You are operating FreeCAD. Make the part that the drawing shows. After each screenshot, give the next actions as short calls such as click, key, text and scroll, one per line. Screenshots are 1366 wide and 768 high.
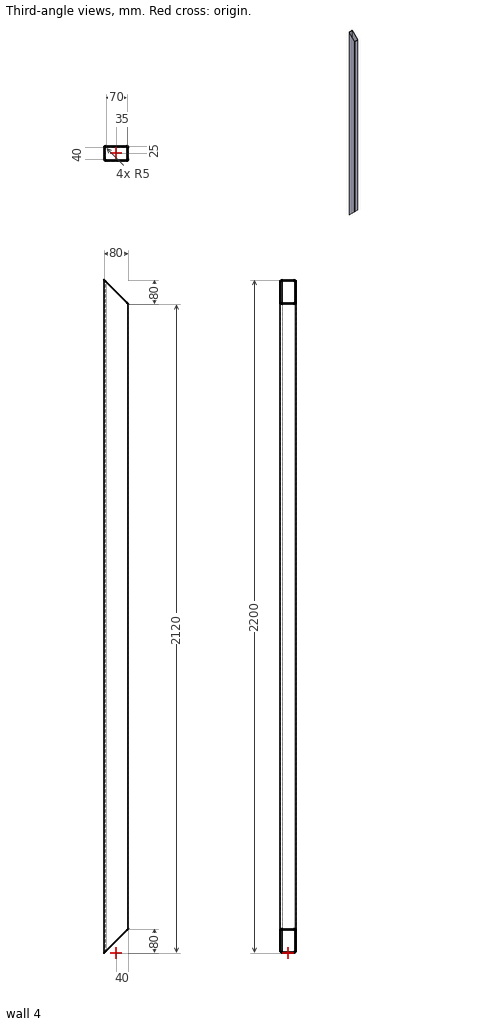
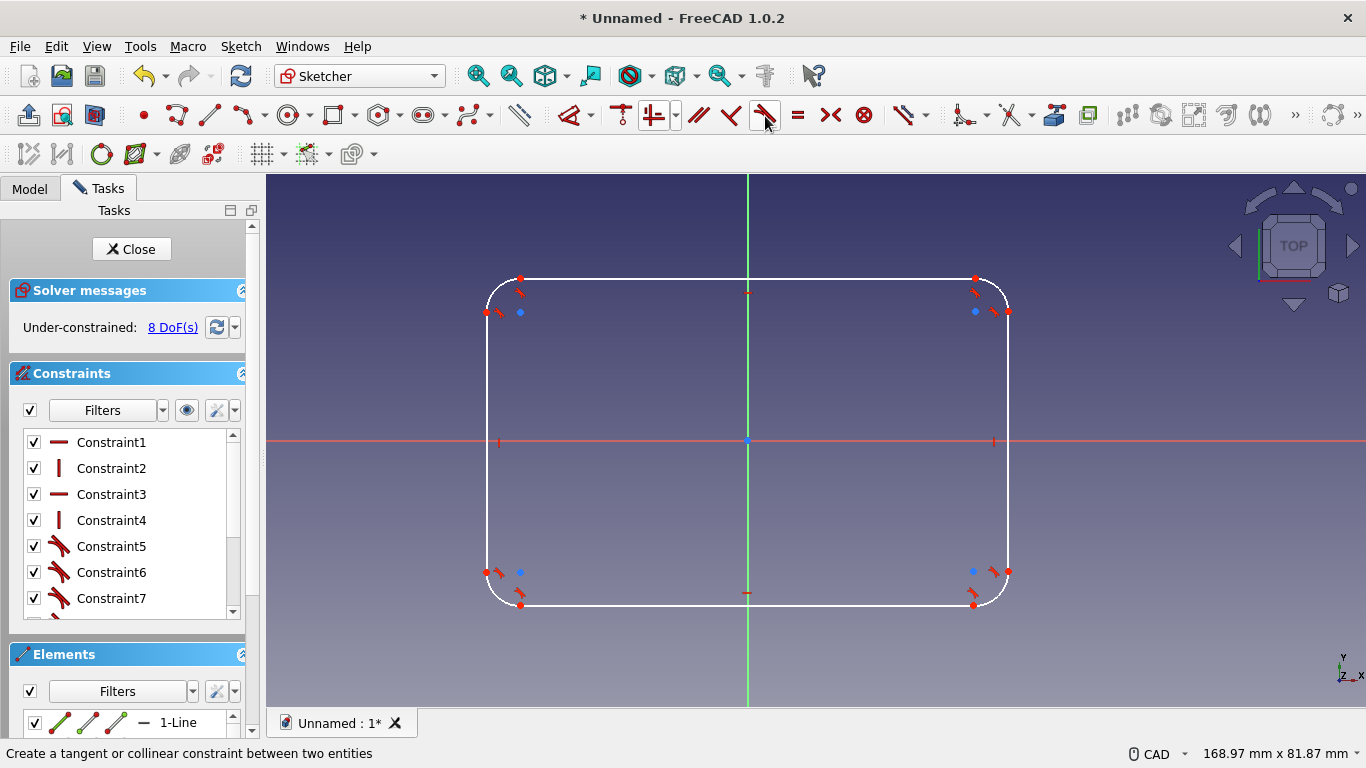
click(505, 283)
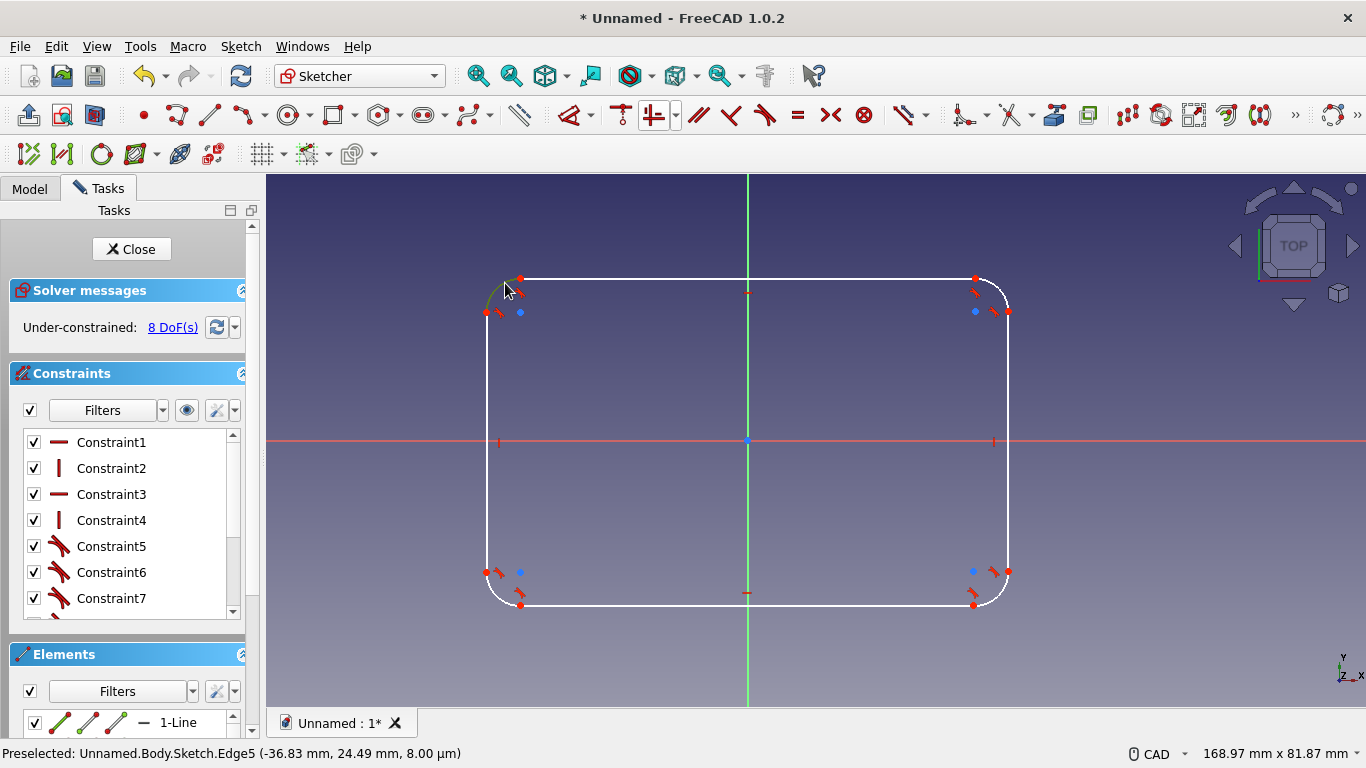
click(490, 588)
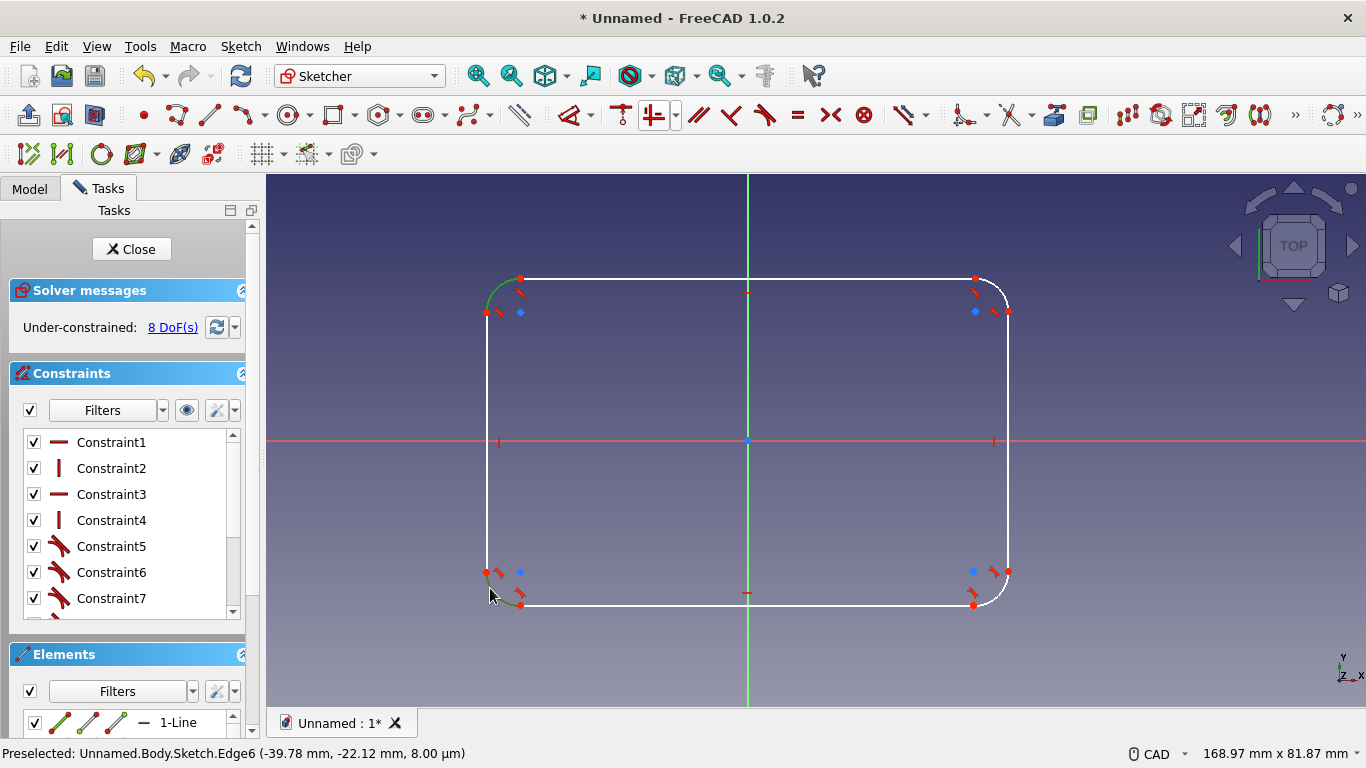
click(990, 602)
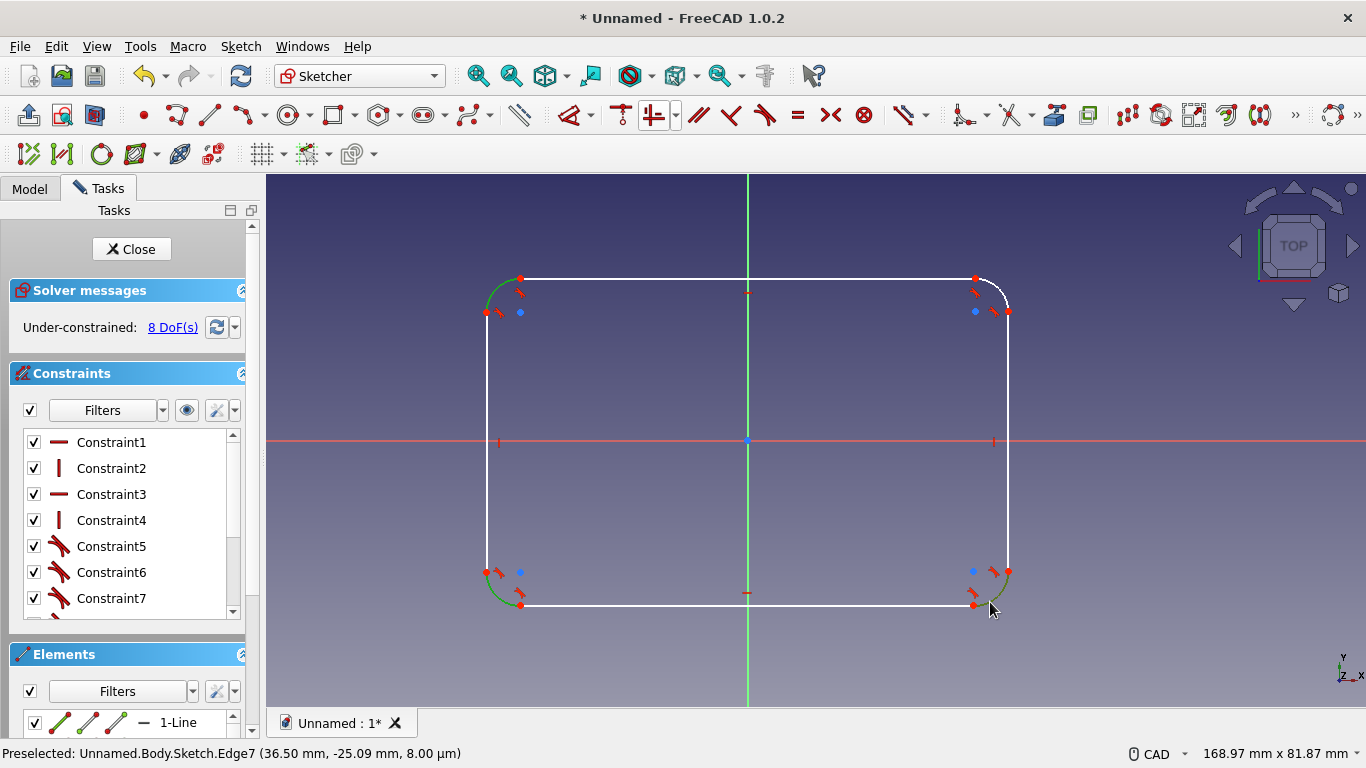
click(1005, 297)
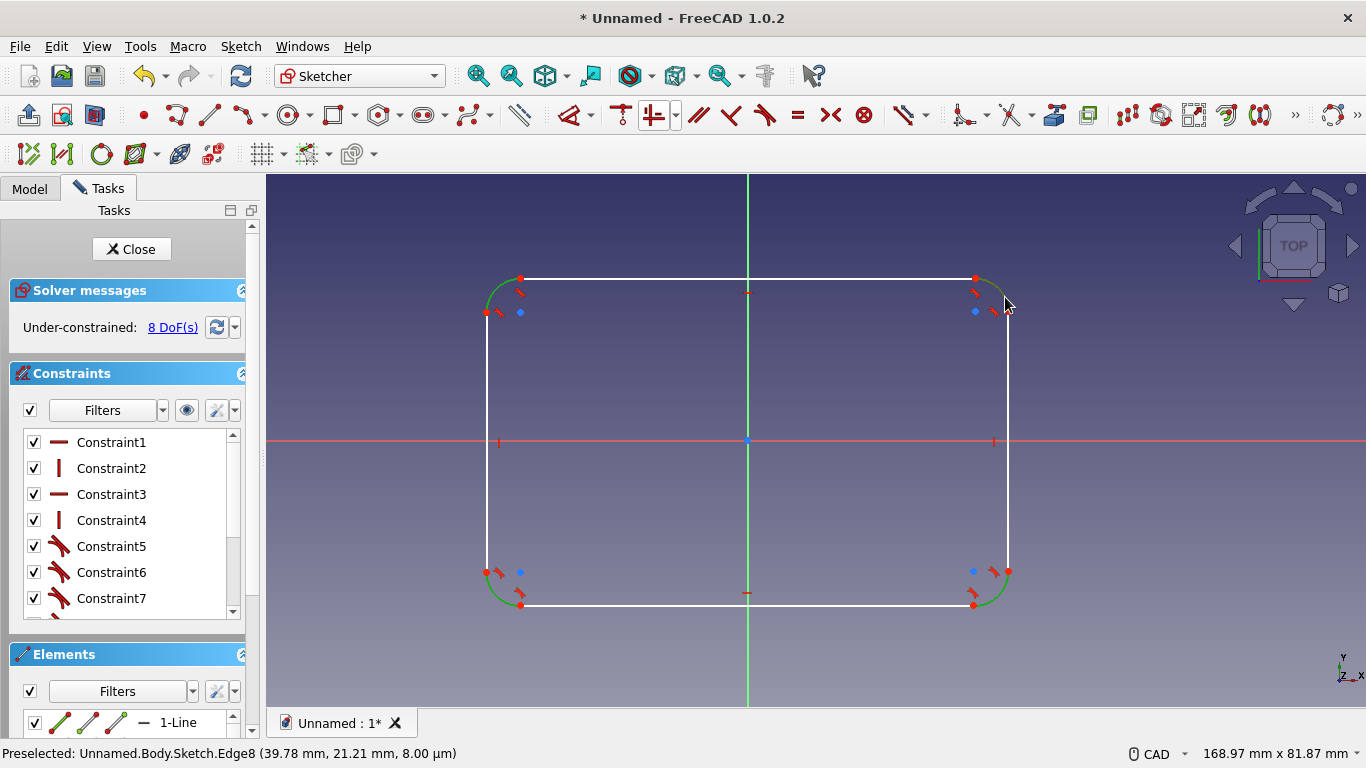
click(798, 116)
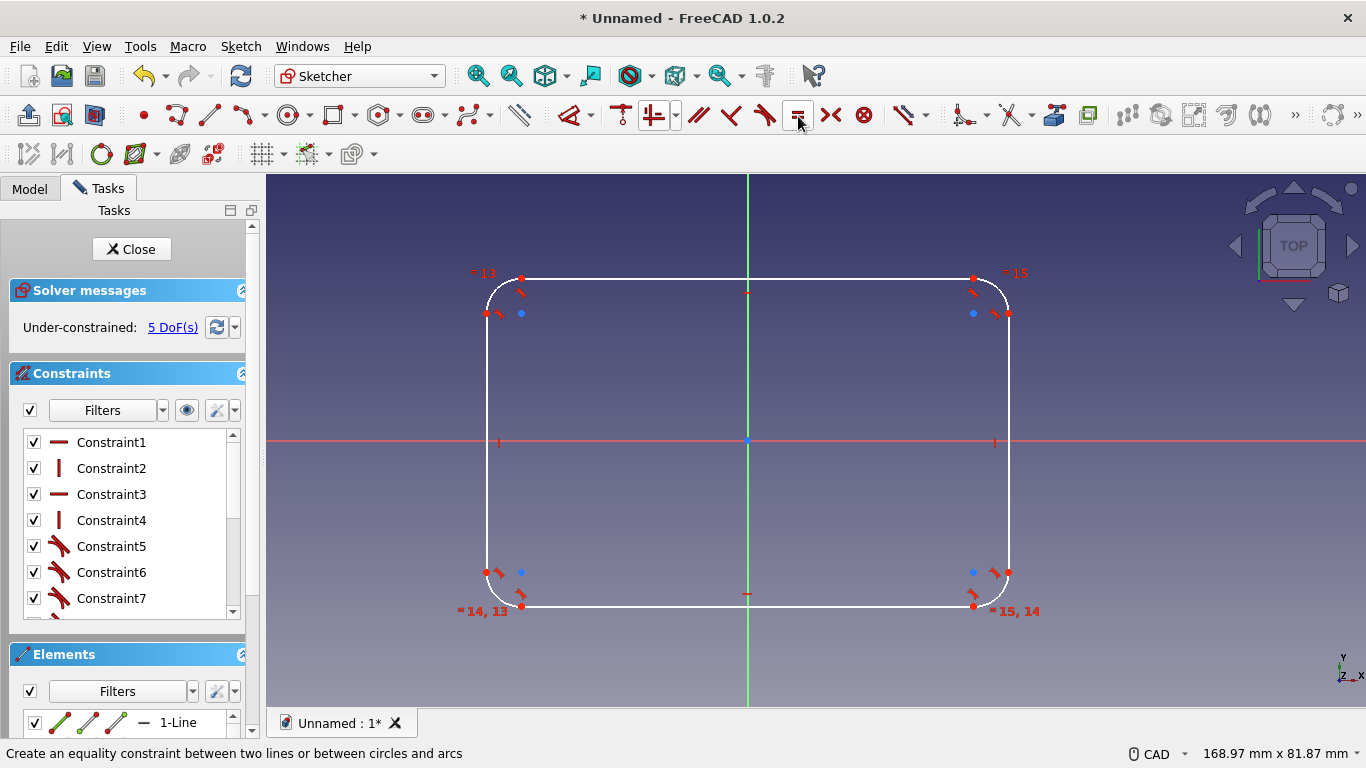
click(568, 116)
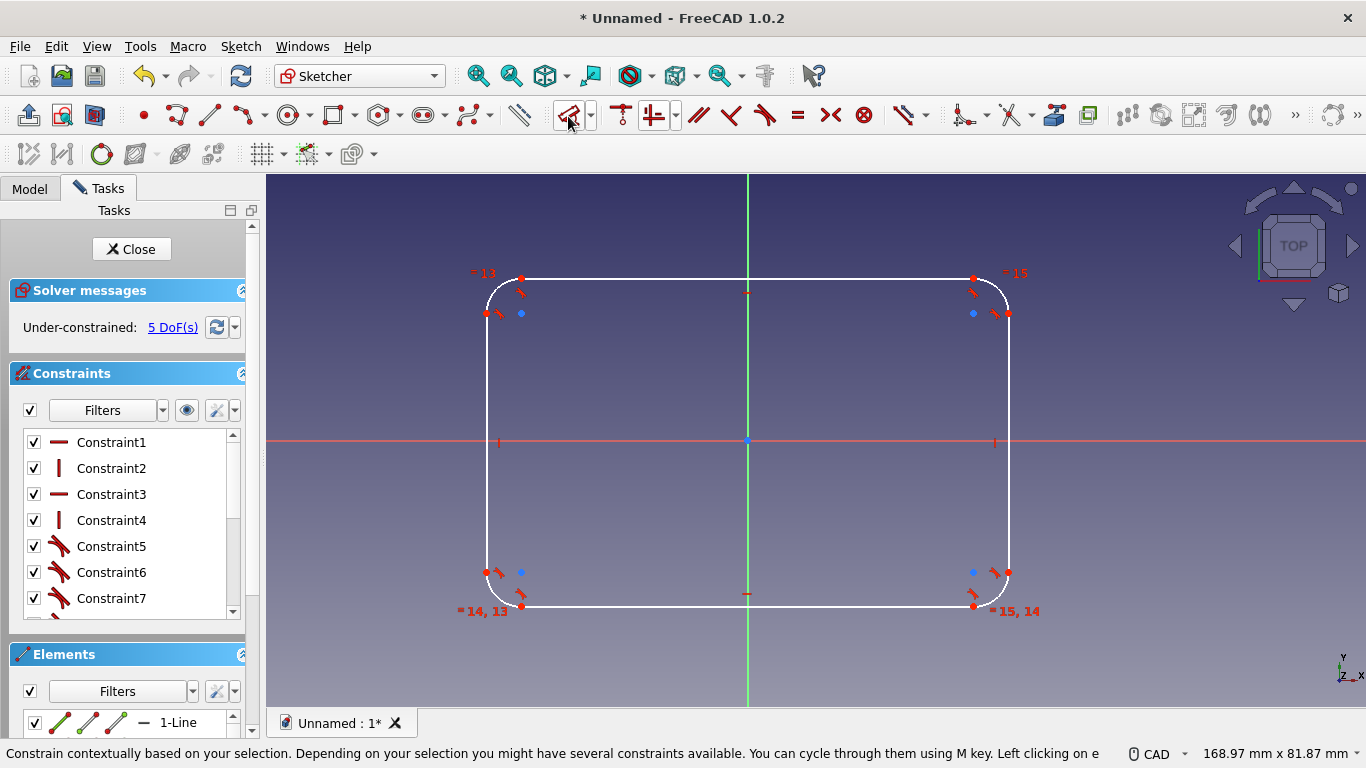
click(506, 283)
click(492, 254)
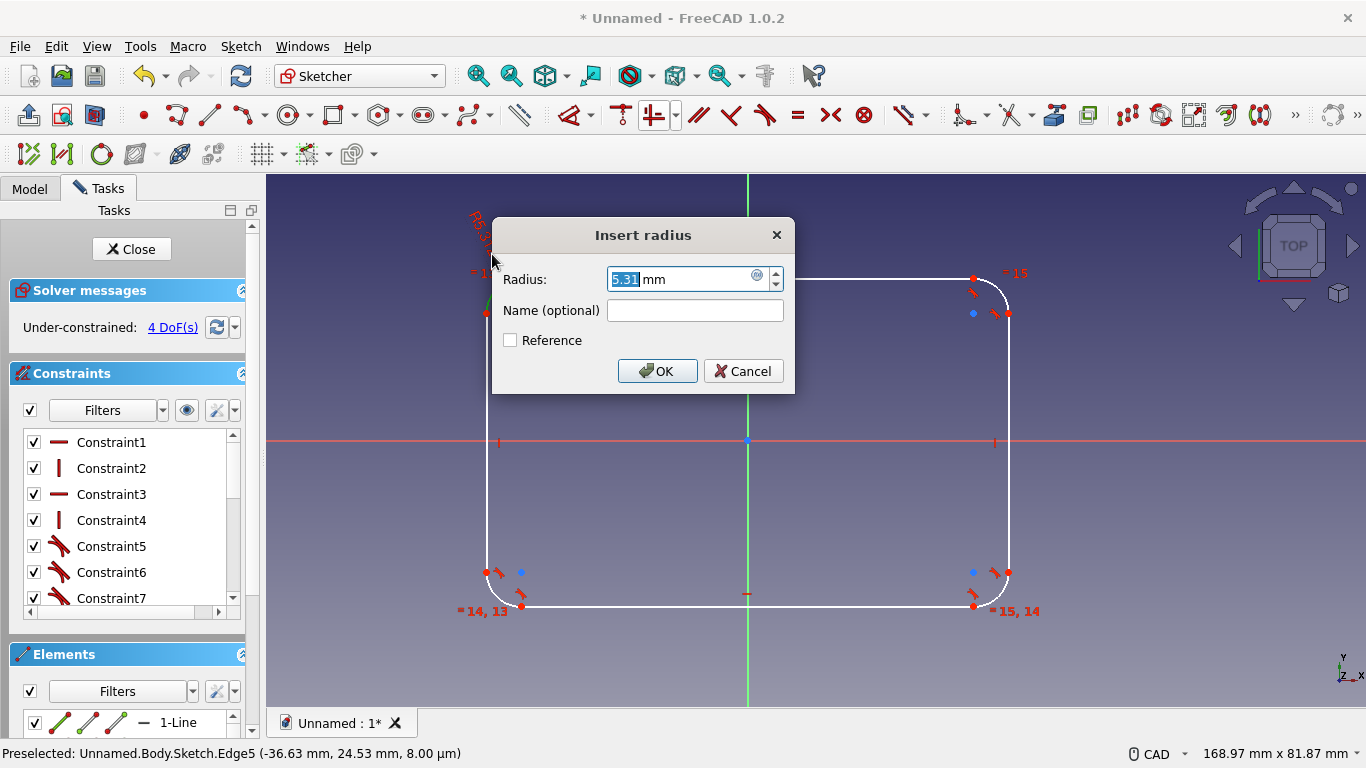
text(5)
key(Return)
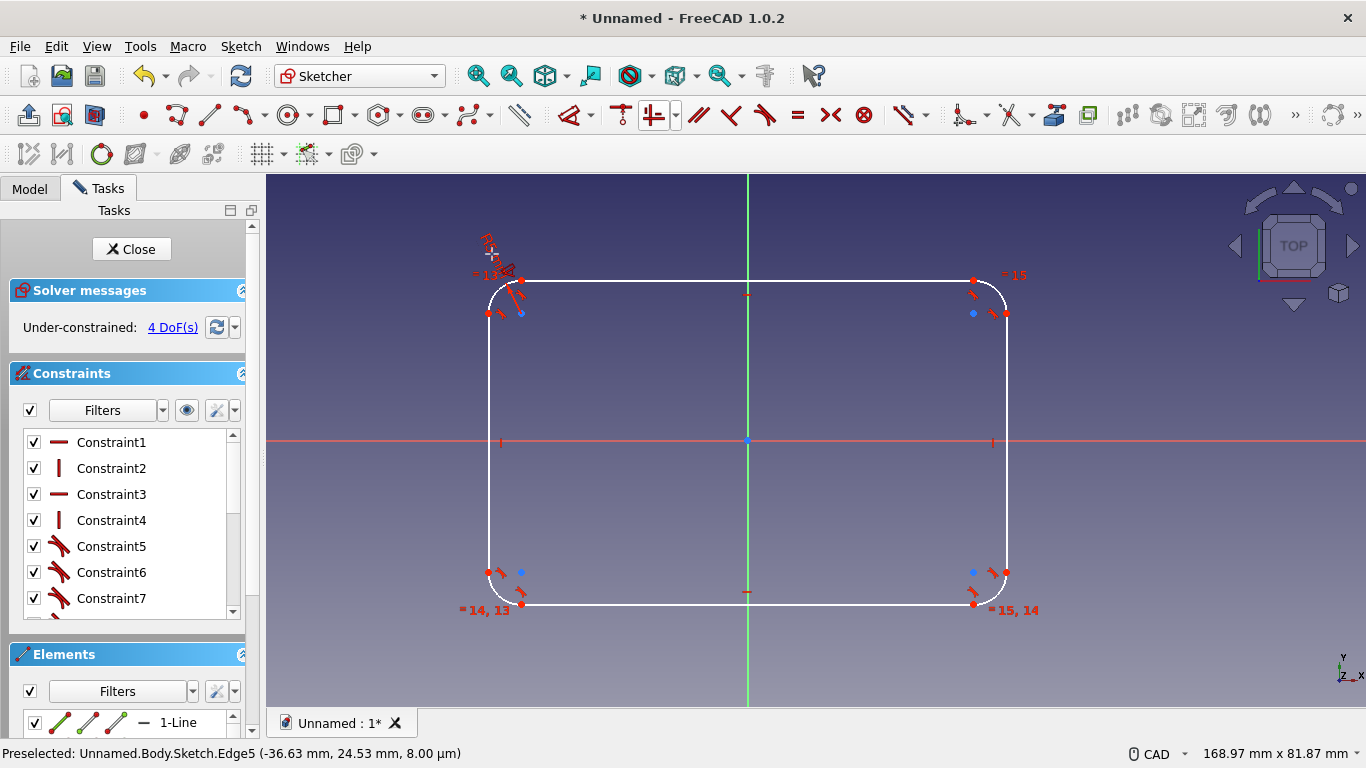
click(838, 281)
click(643, 247)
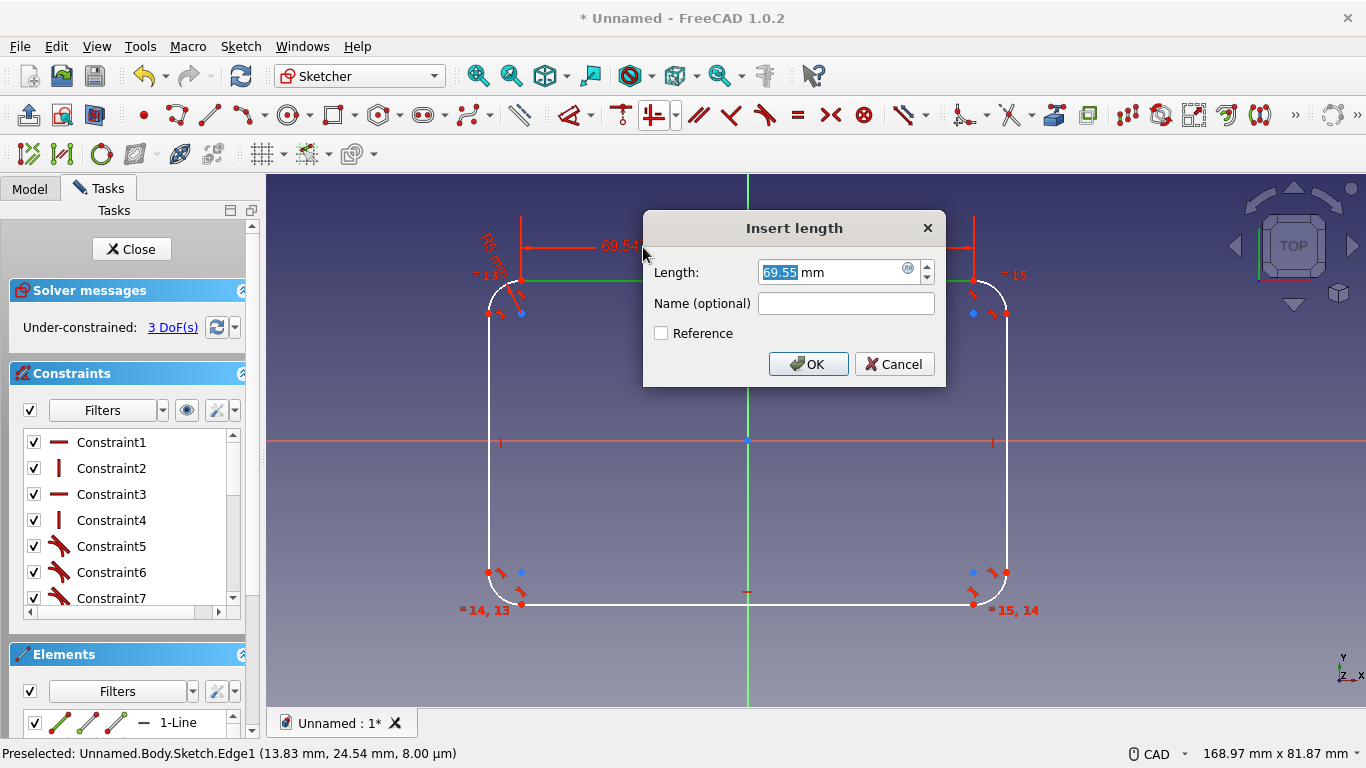
text(70)
key(Return)